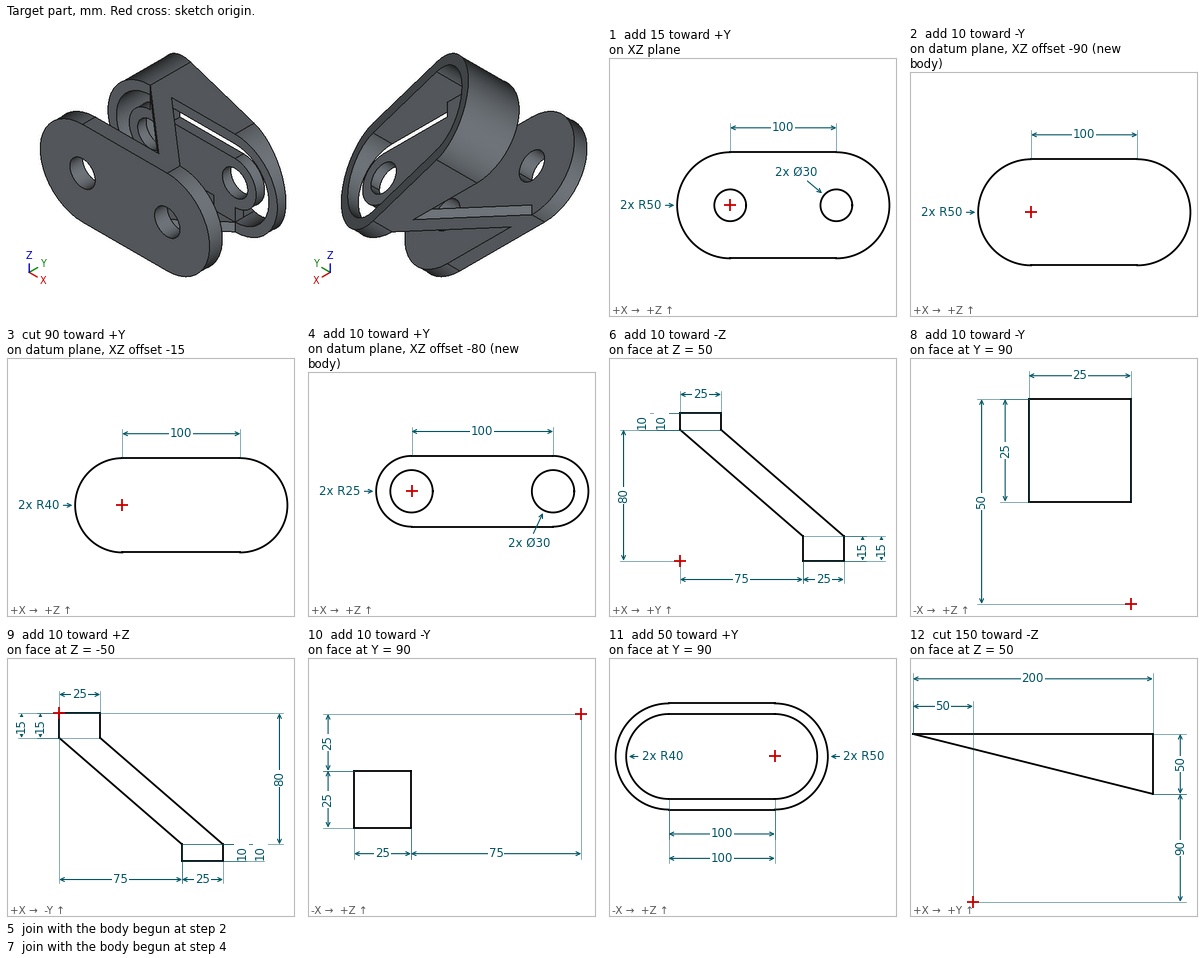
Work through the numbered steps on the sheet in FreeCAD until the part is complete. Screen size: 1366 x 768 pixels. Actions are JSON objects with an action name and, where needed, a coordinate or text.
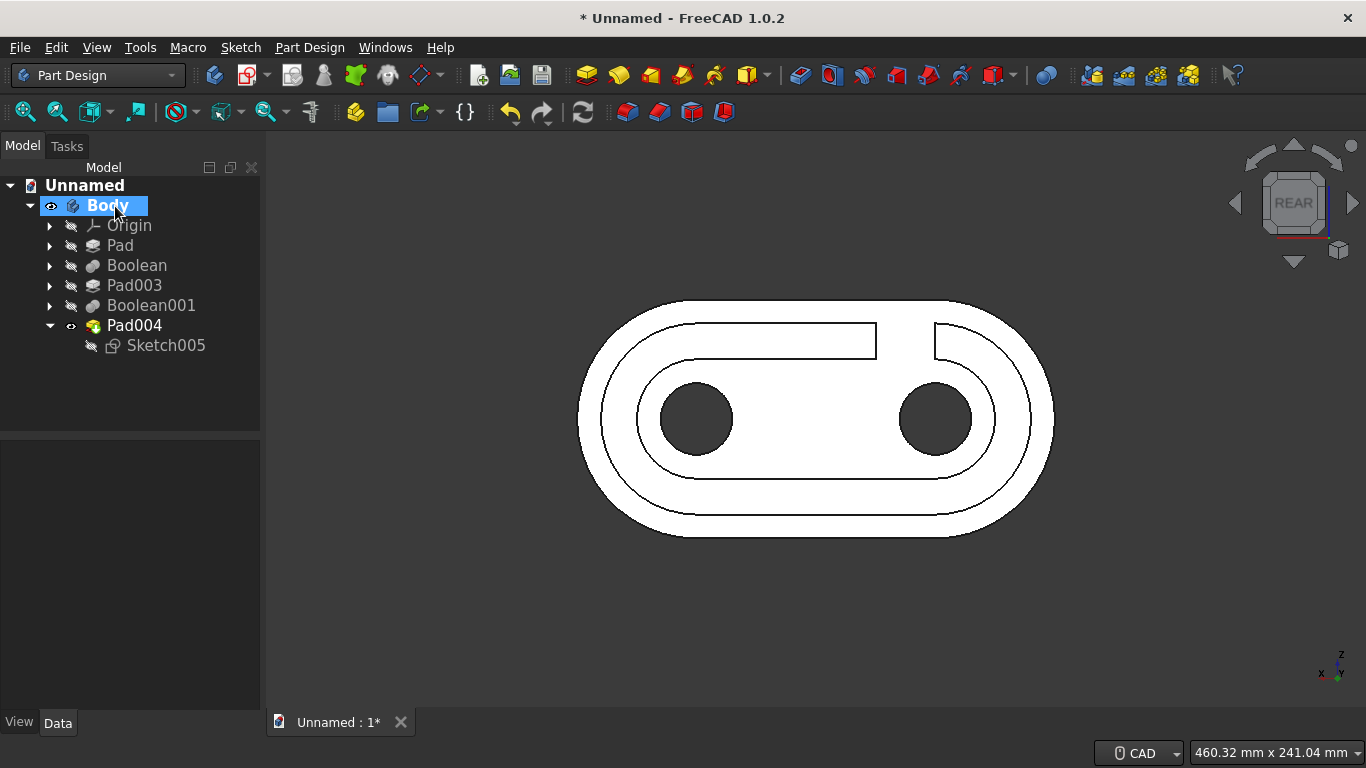
{"action": "left_click", "coordinate": [26, 112]}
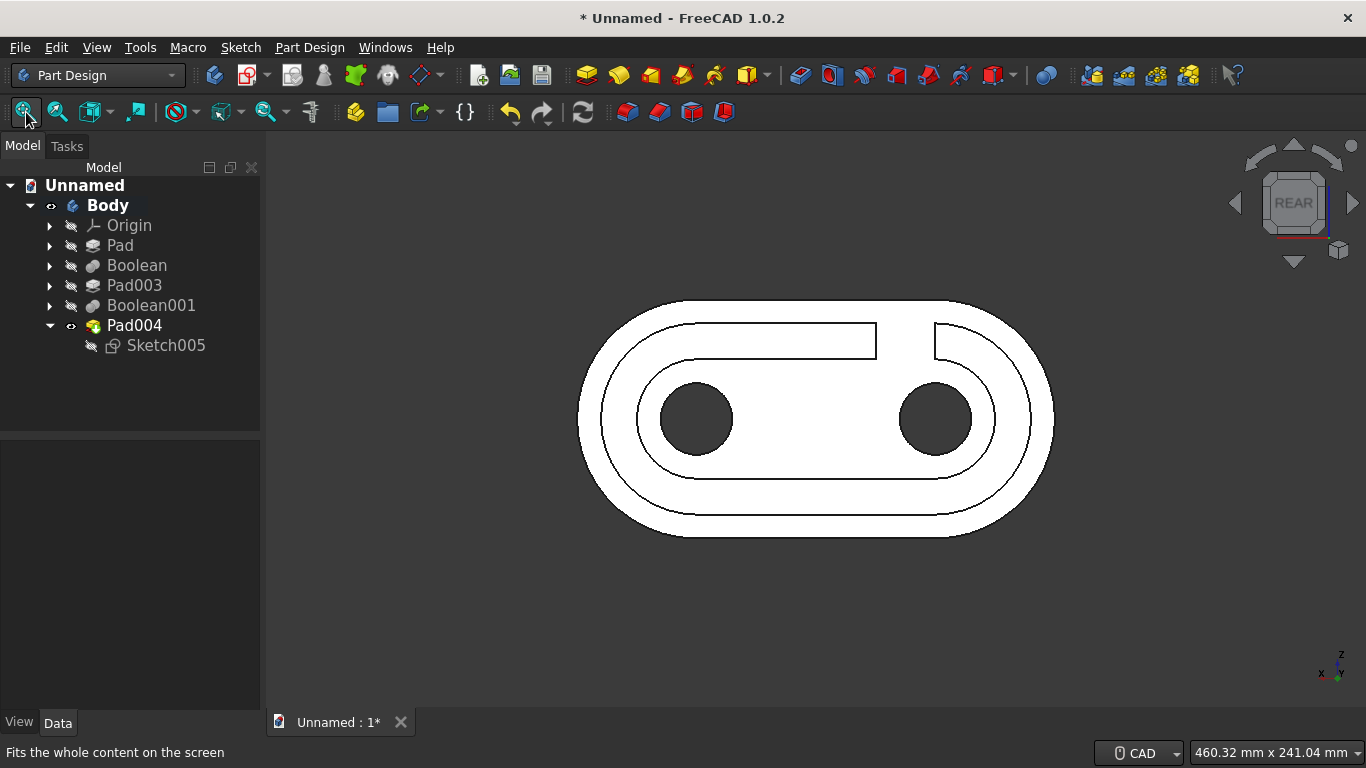
{"action": "key", "text": "5"}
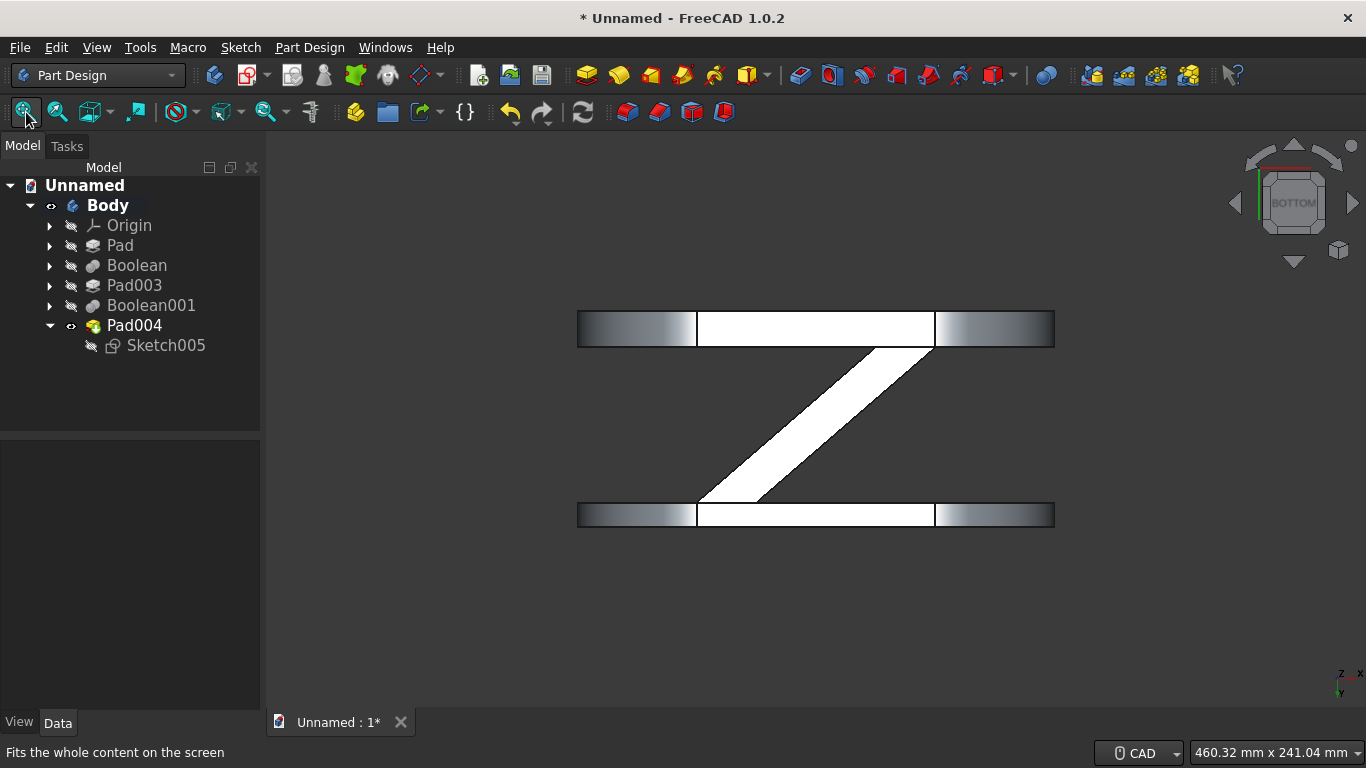
{"action": "left_click", "coordinate": [26, 112]}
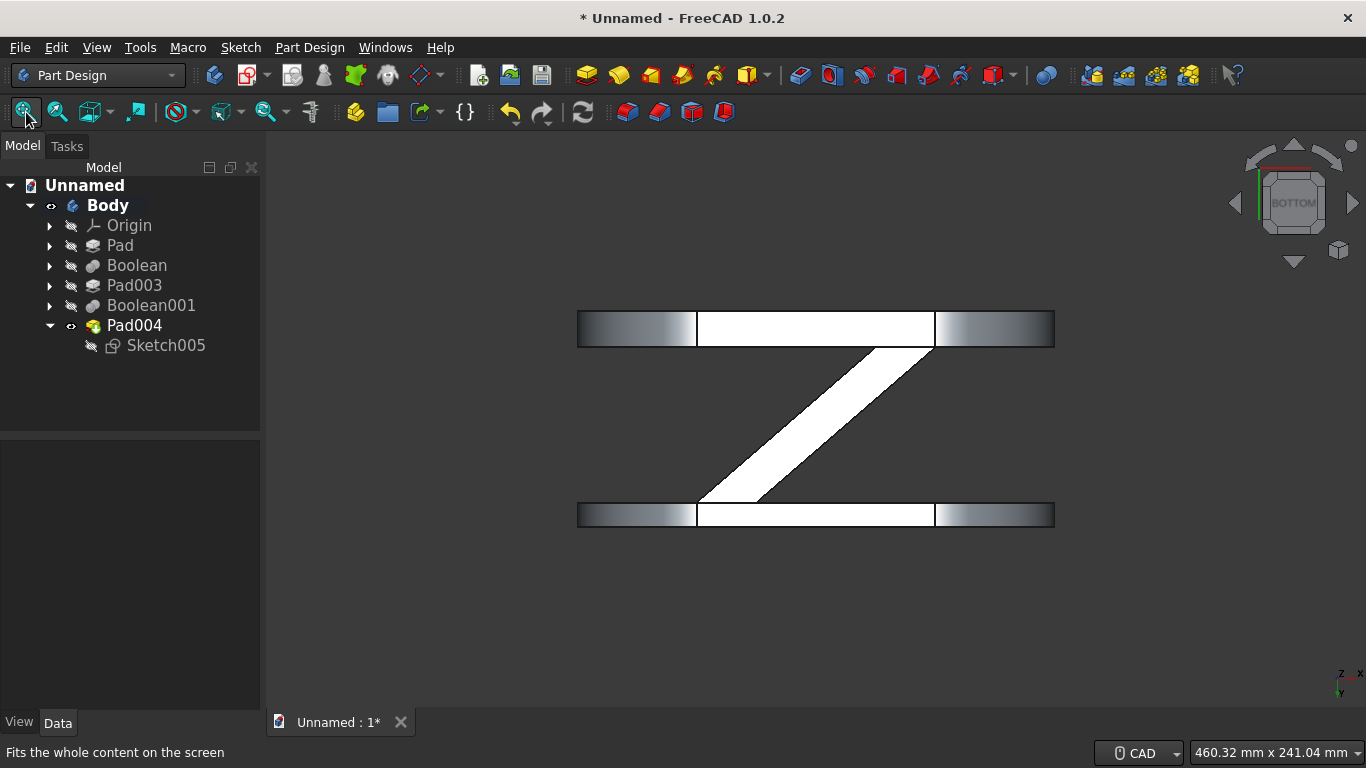
{"action": "left_click", "coordinate": [884, 328]}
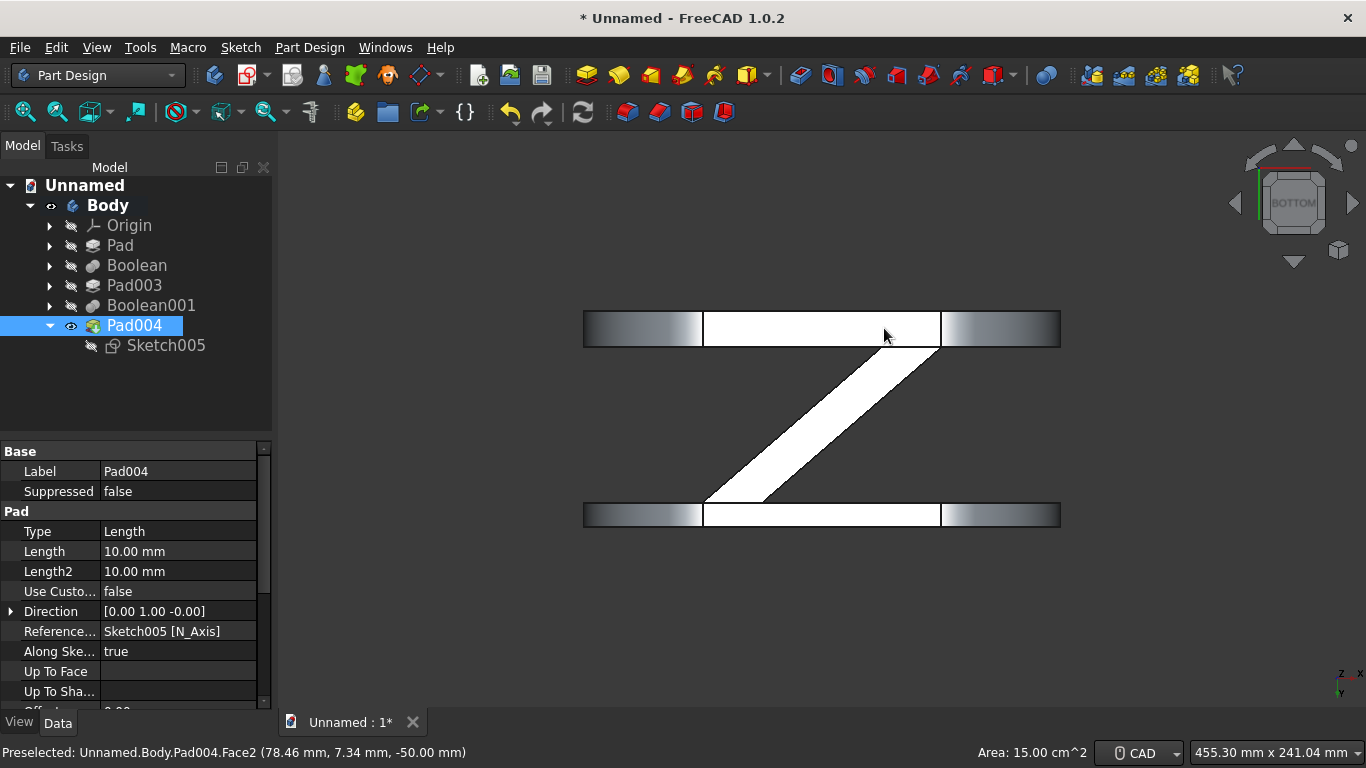
{"action": "left_click", "coordinate": [248, 76]}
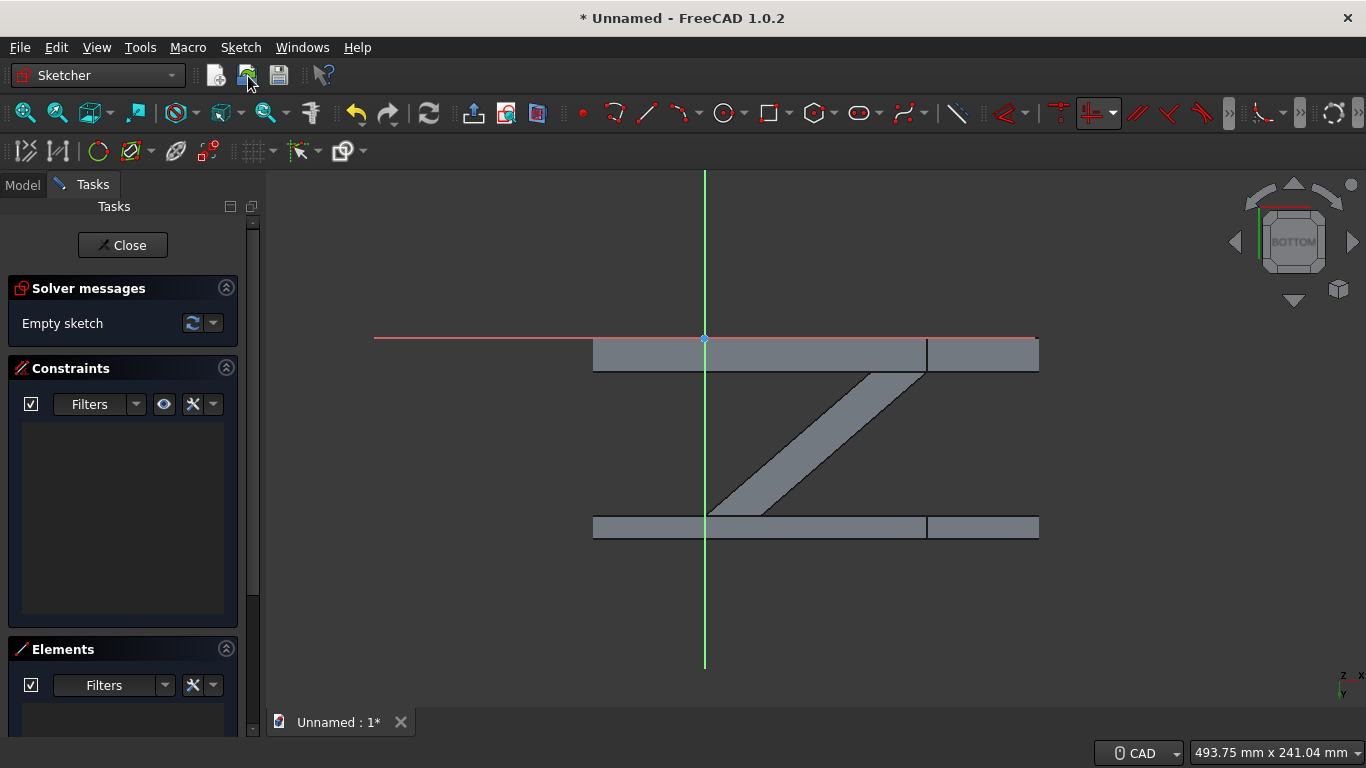
{"action": "scroll", "coordinate": [899, 438], "scroll_direction": "up", "scroll_amount": 3}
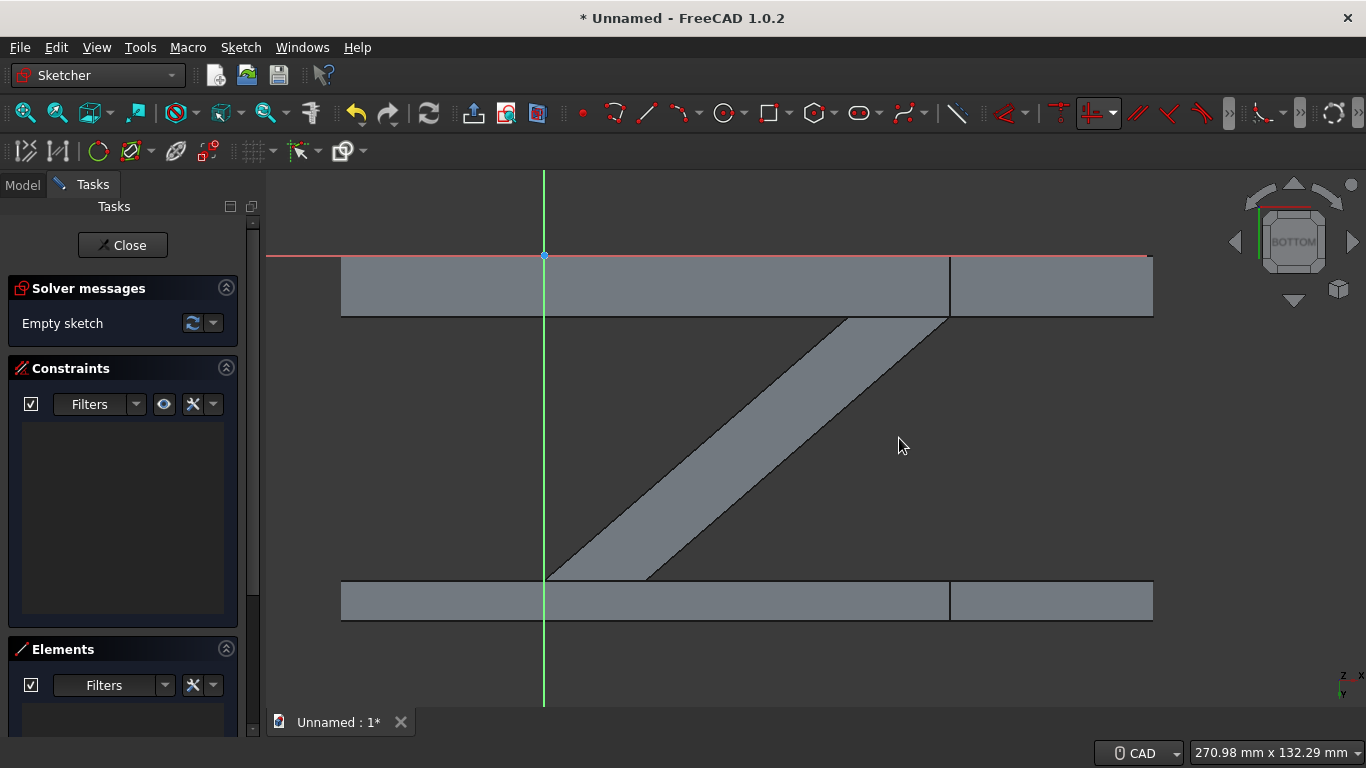
{"action": "left_click", "coordinate": [616, 114]}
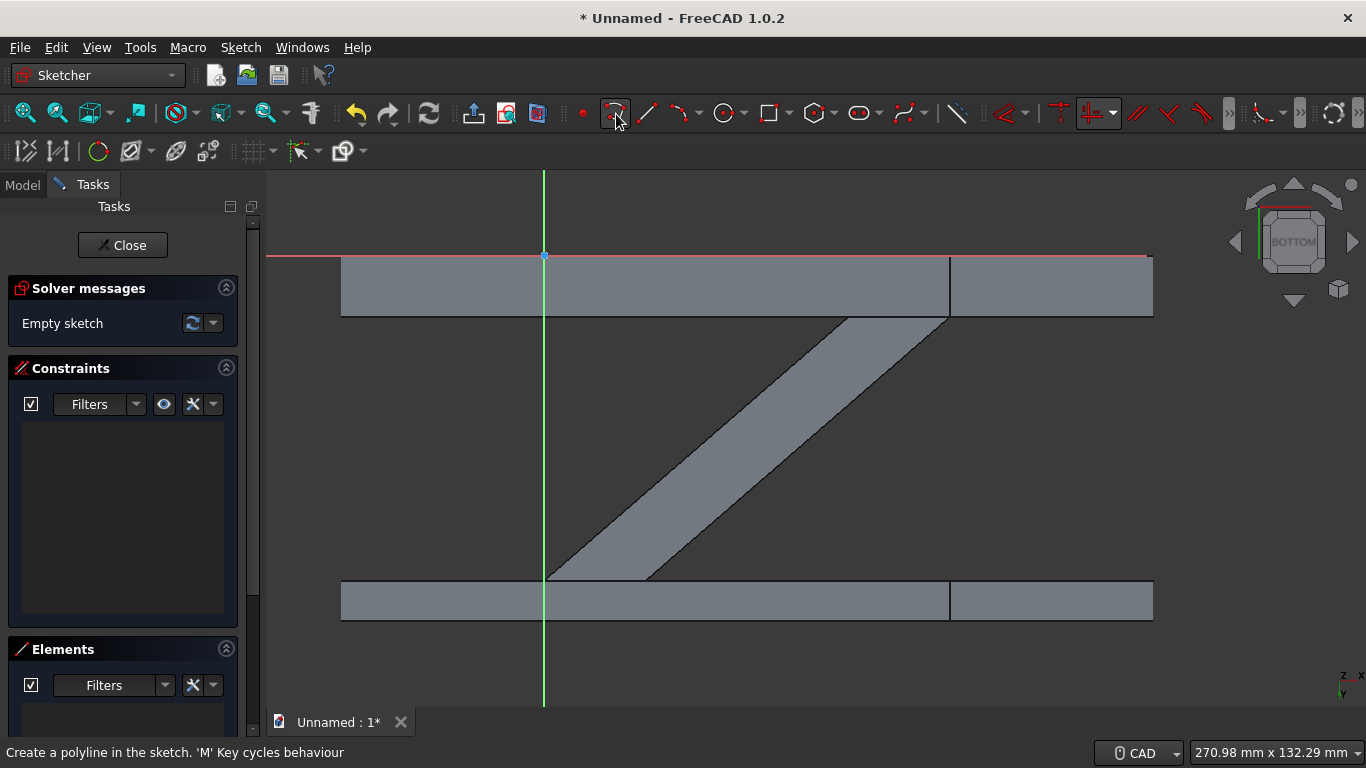
{"action": "left_click", "coordinate": [544, 256]}
{"action": "left_click", "coordinate": [553, 317]}
{"action": "left_click", "coordinate": [849, 581]}
{"action": "left_click", "coordinate": [849, 621]}
{"action": "left_click", "coordinate": [950, 621]}
{"action": "left_click", "coordinate": [950, 581]}
{"action": "left_click", "coordinate": [646, 317]}
{"action": "left_click", "coordinate": [646, 265]}
{"action": "left_click", "coordinate": [544, 256]}
{"action": "key", "text": "Escape"}
{"action": "key", "text": "Escape"}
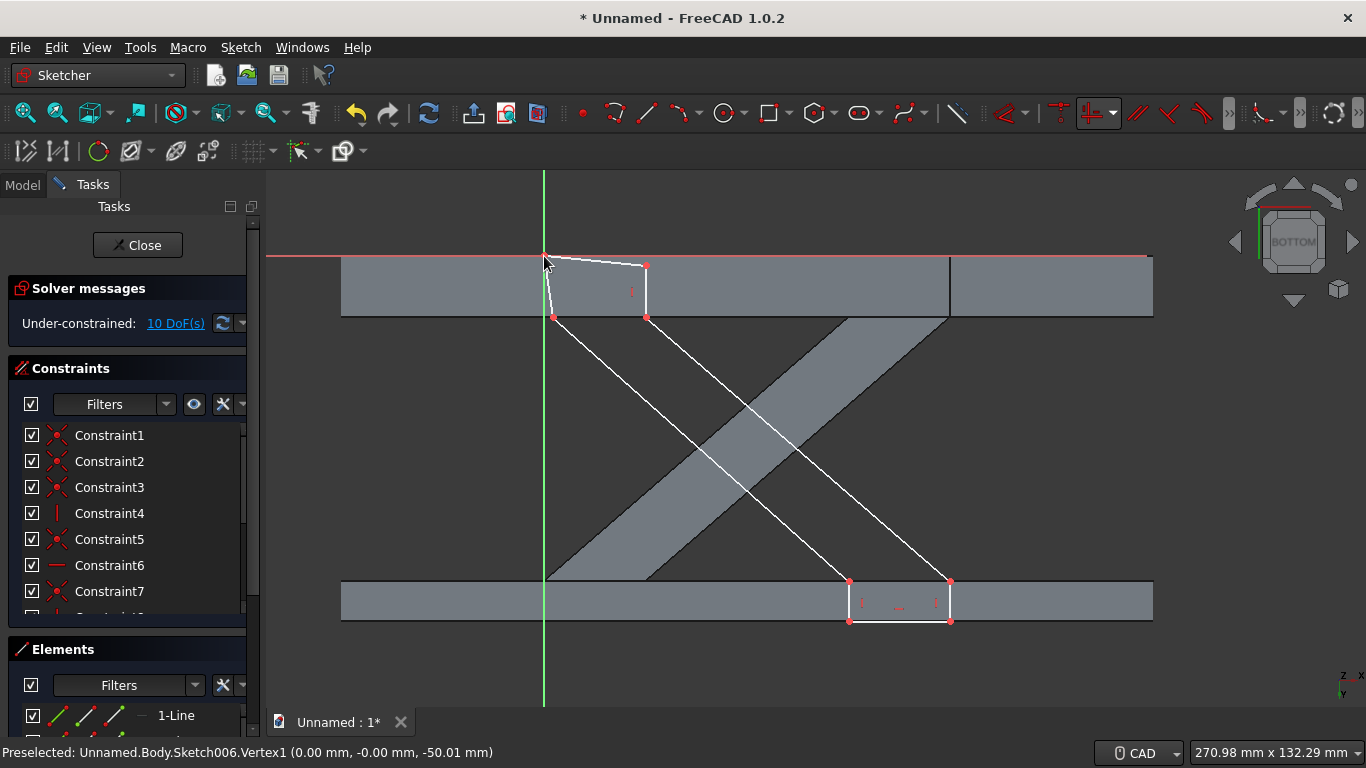
{"action": "left_click", "coordinate": [547, 274]}